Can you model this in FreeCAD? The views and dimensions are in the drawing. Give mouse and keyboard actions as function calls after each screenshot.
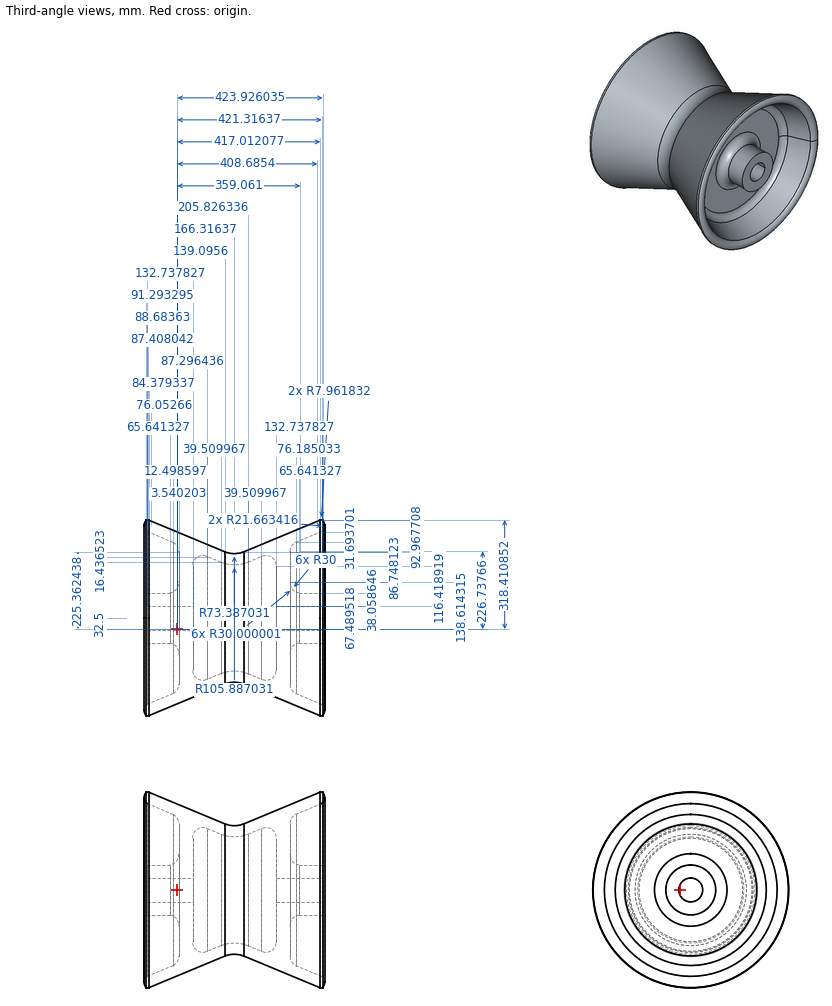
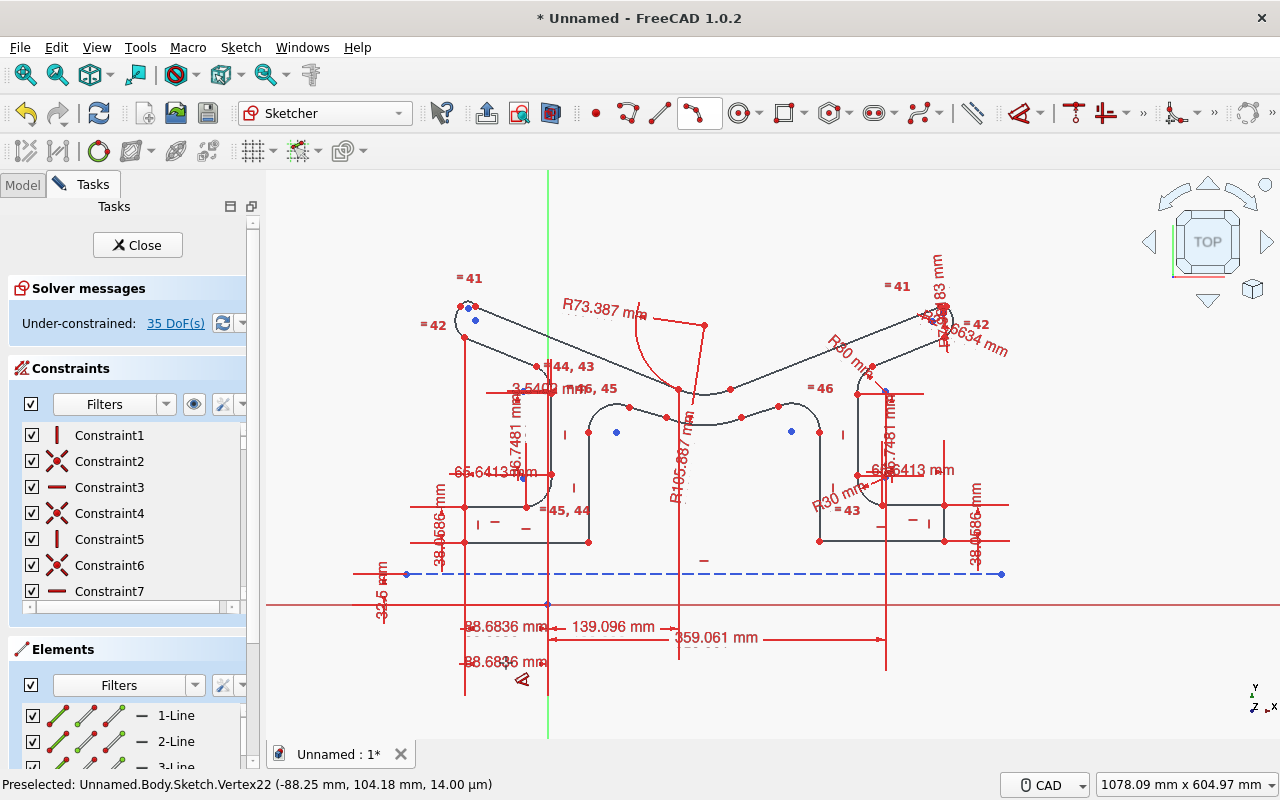
click(933, 321)
click(829, 639)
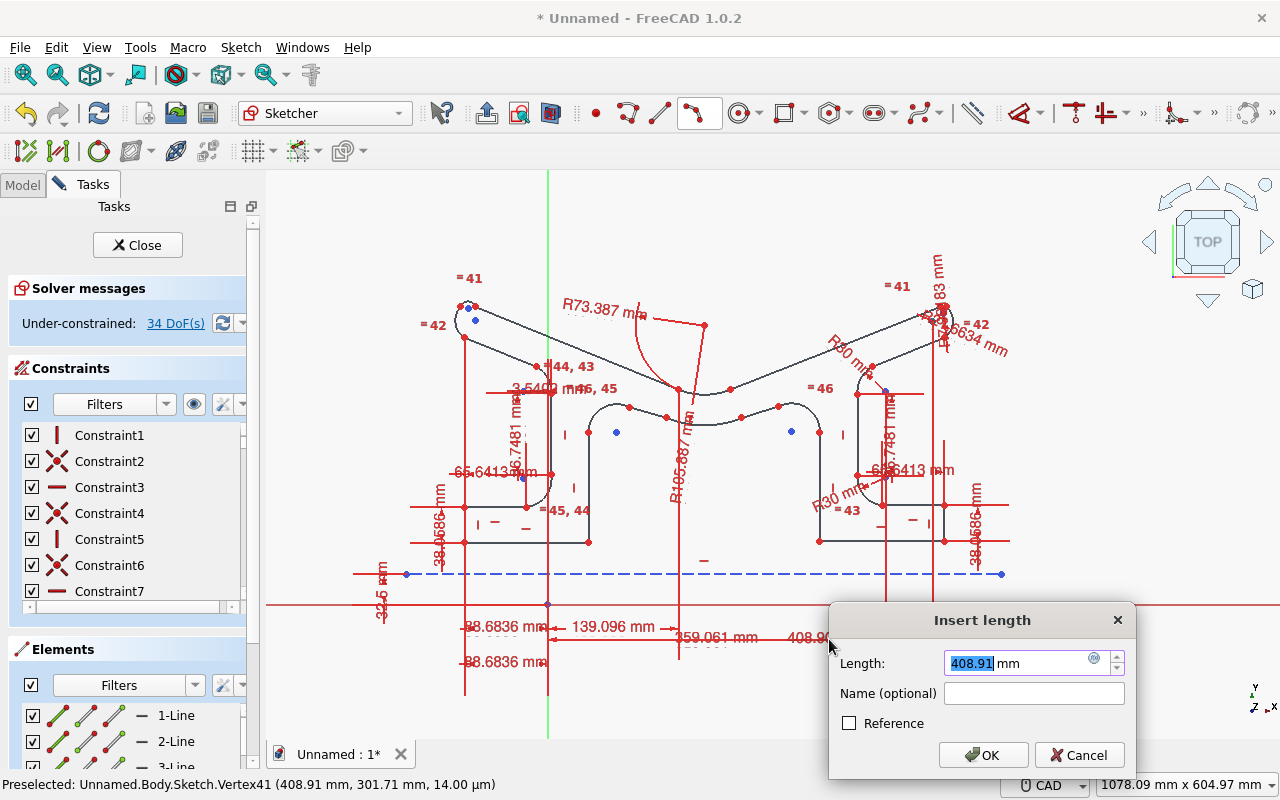
text(408.6854)
key(Return)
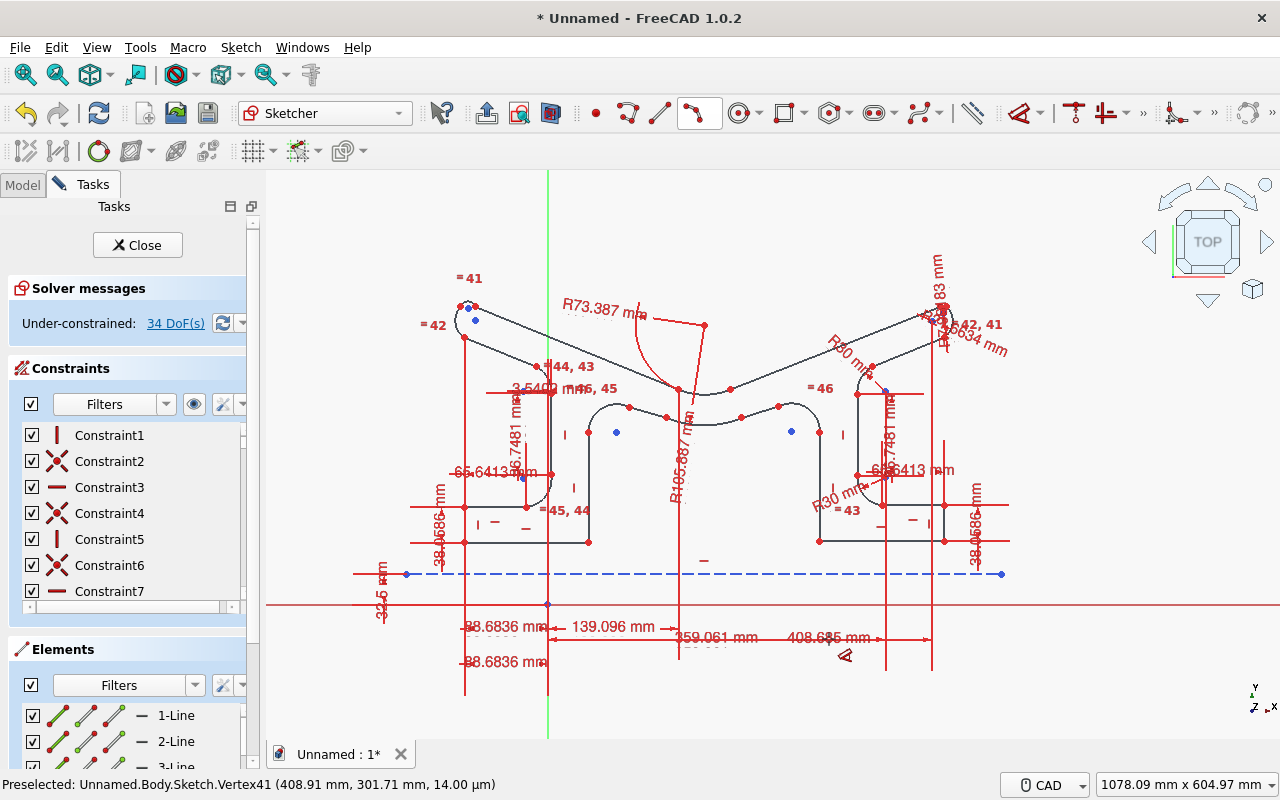
click(476, 321)
click(512, 287)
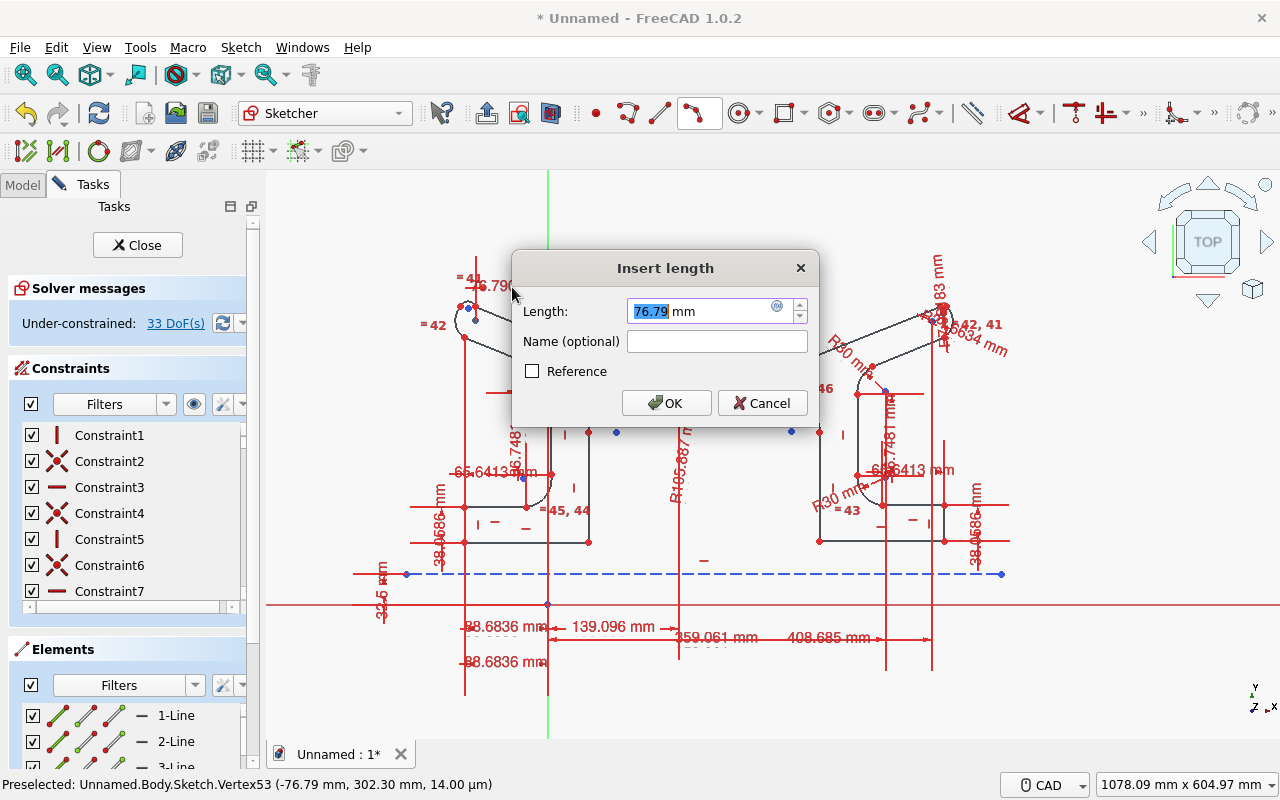
text(76.05266)
key(Return)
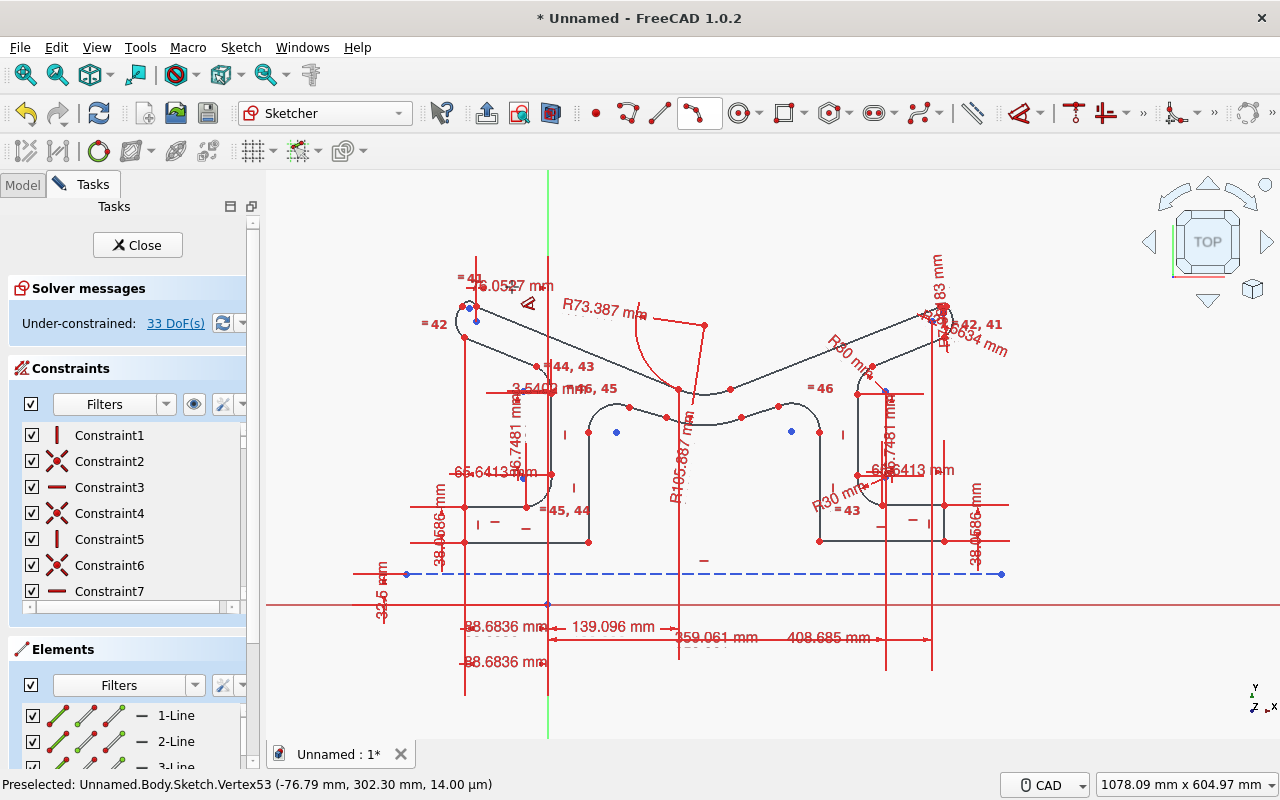
click(820, 465)
click(854, 525)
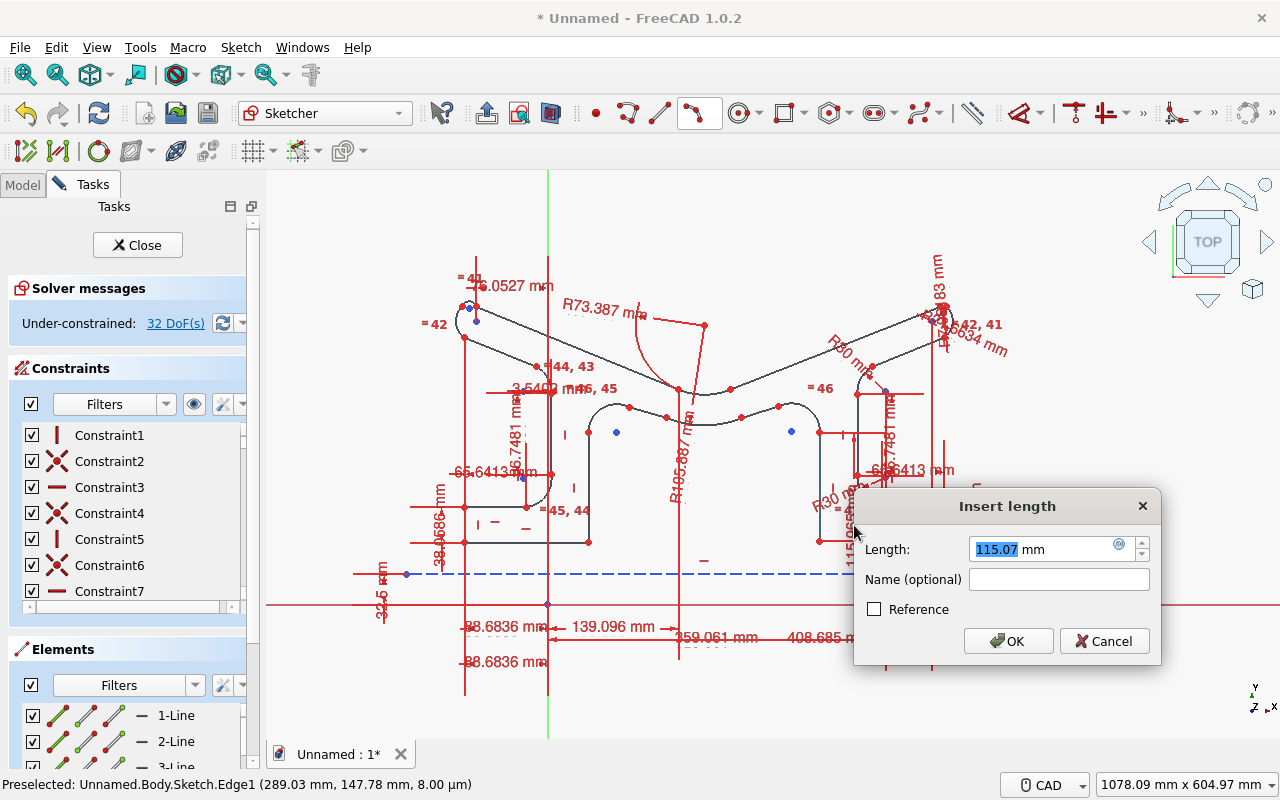
text(116.418919)
key(Return)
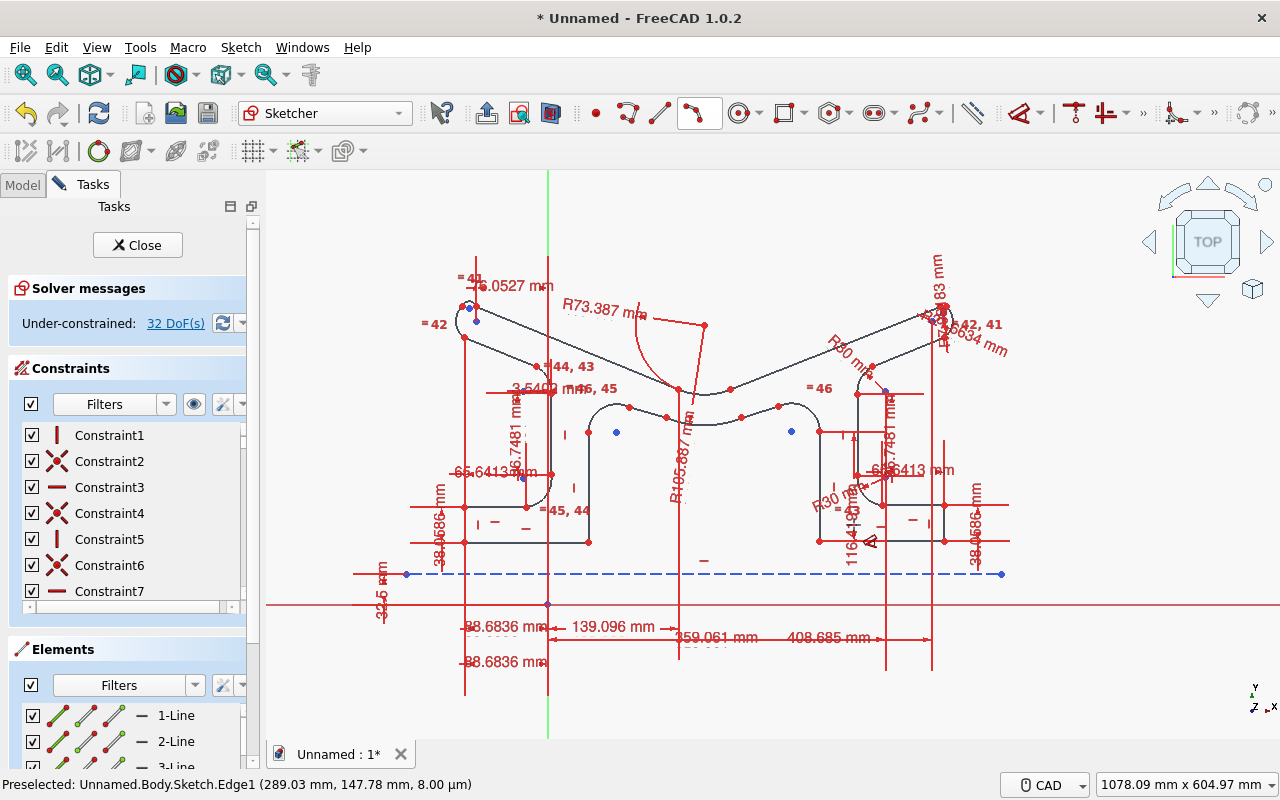
click(857, 541)
click(911, 623)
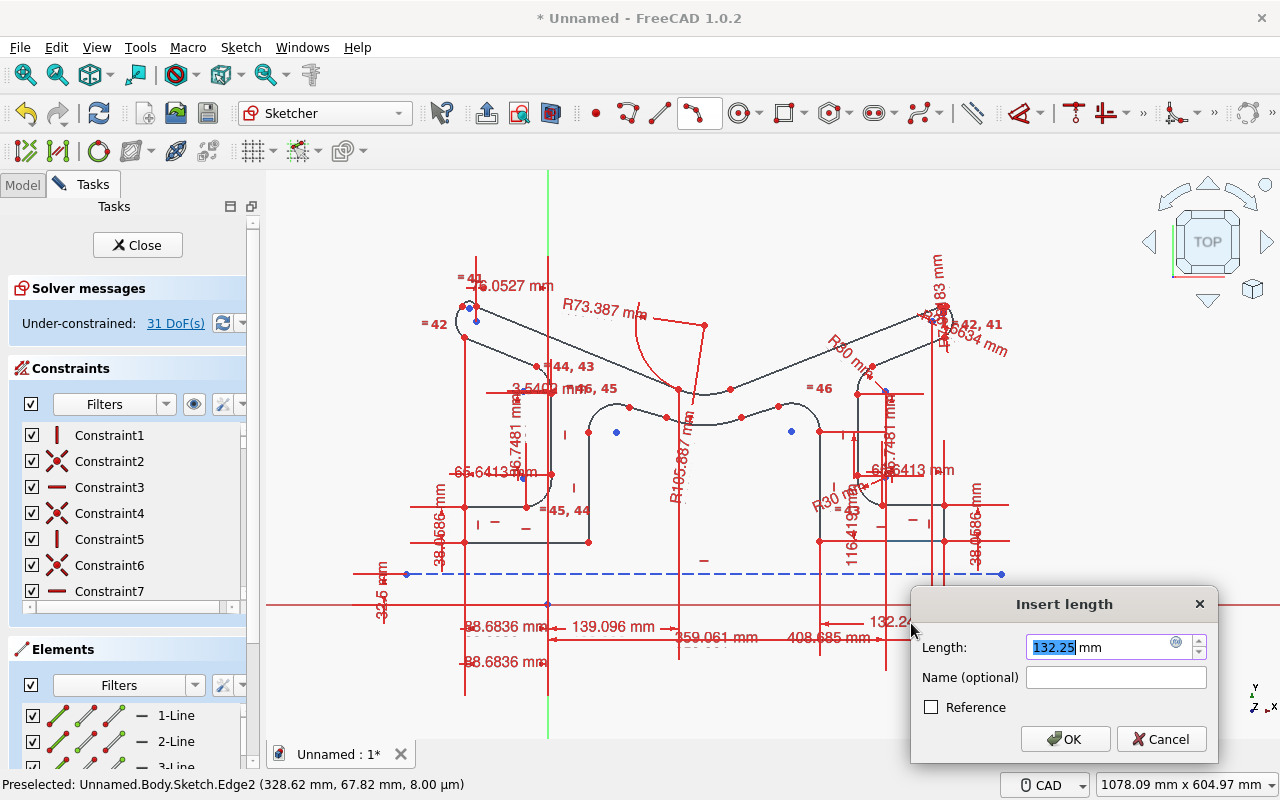
text(132.737827)
key(Return)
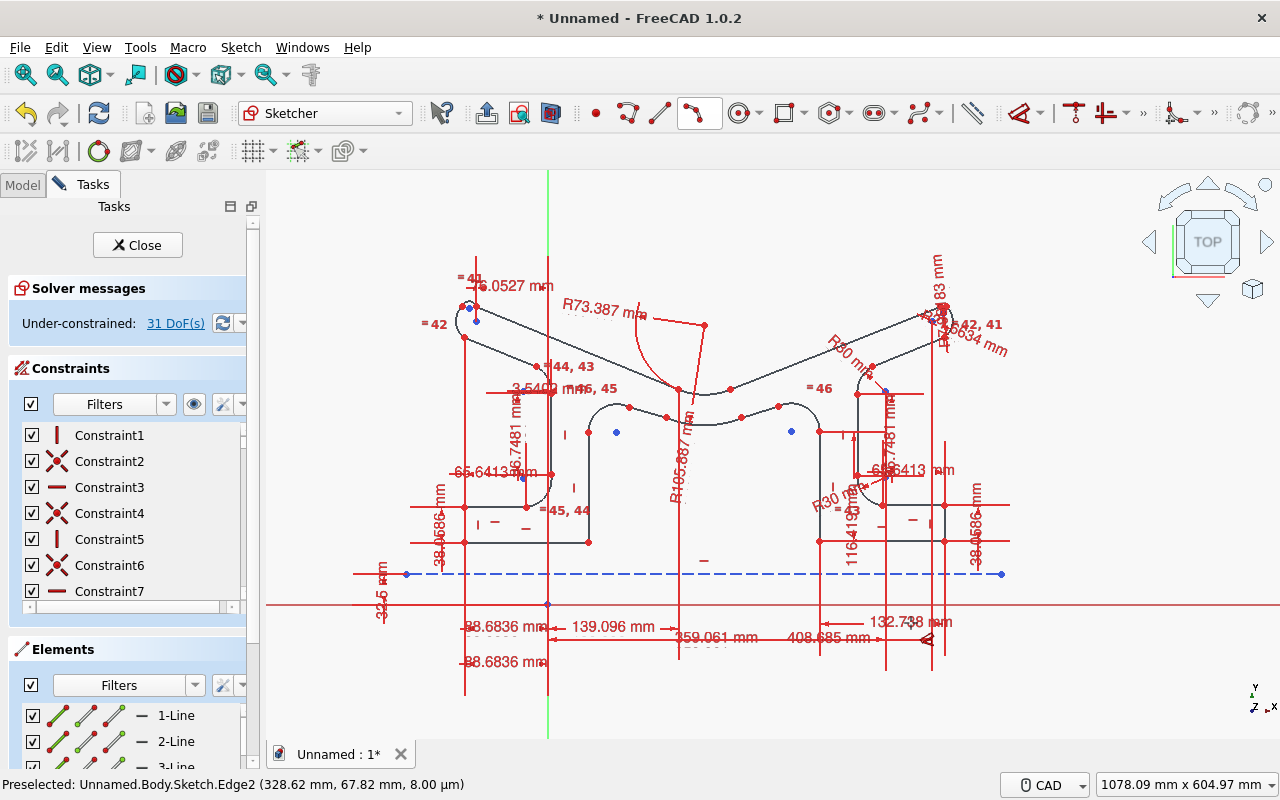
click(502, 543)
click(570, 509)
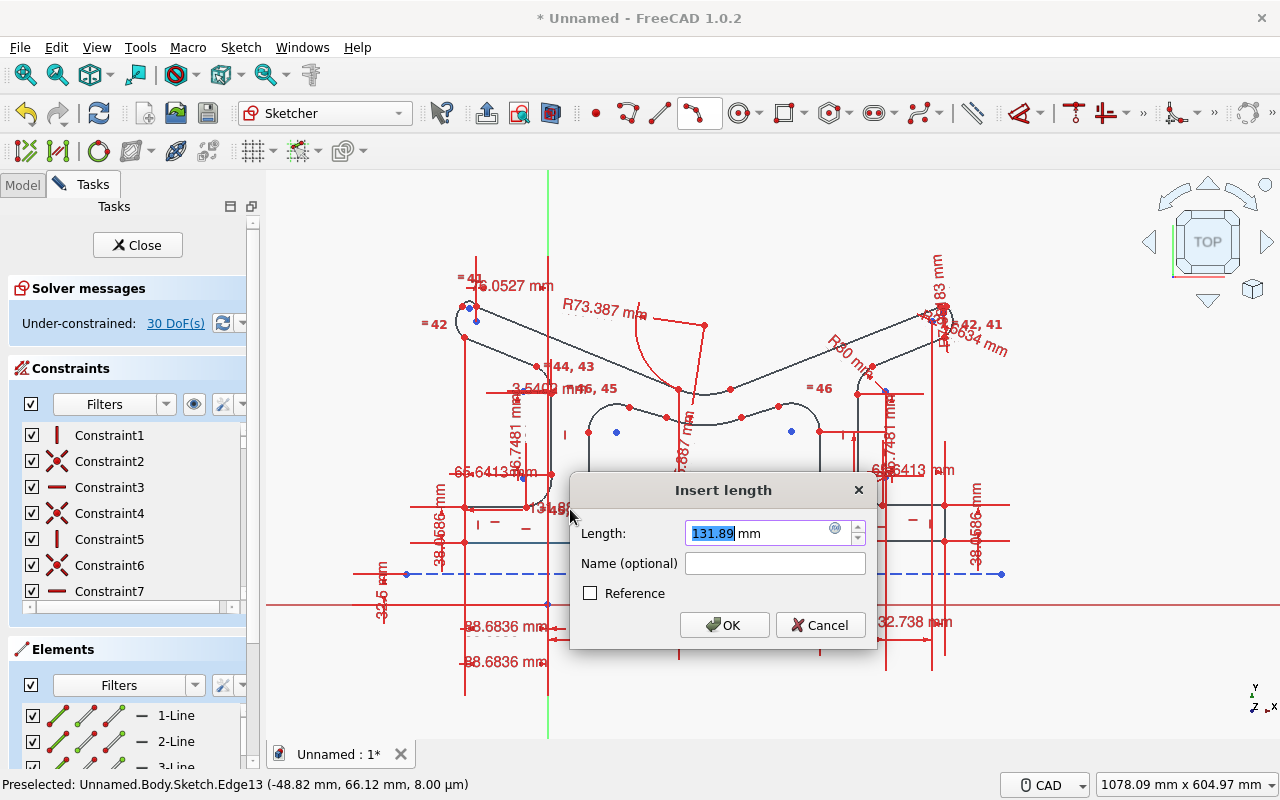
text(132.737827)
key(Return)